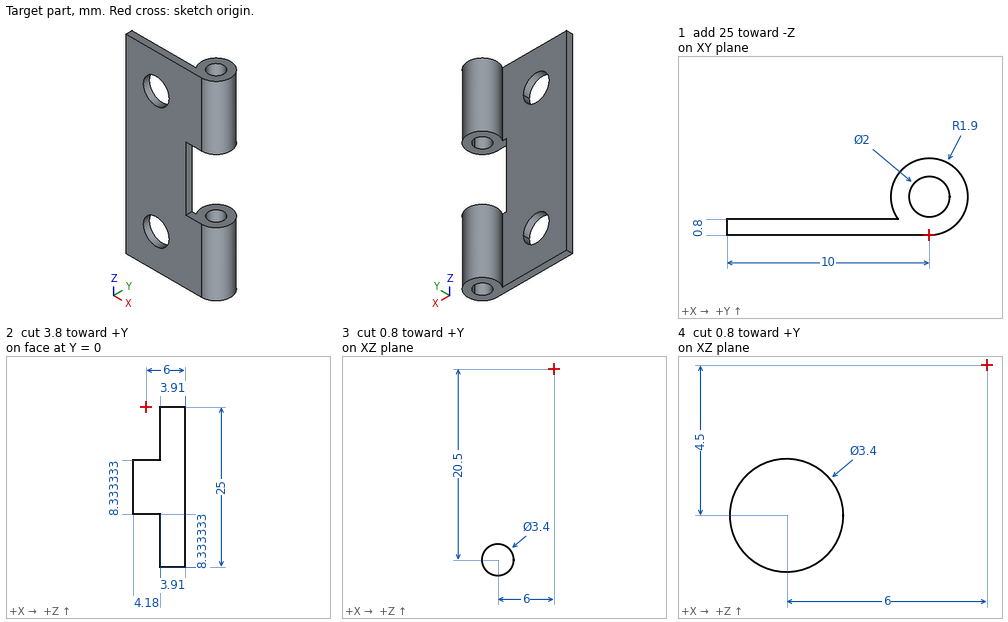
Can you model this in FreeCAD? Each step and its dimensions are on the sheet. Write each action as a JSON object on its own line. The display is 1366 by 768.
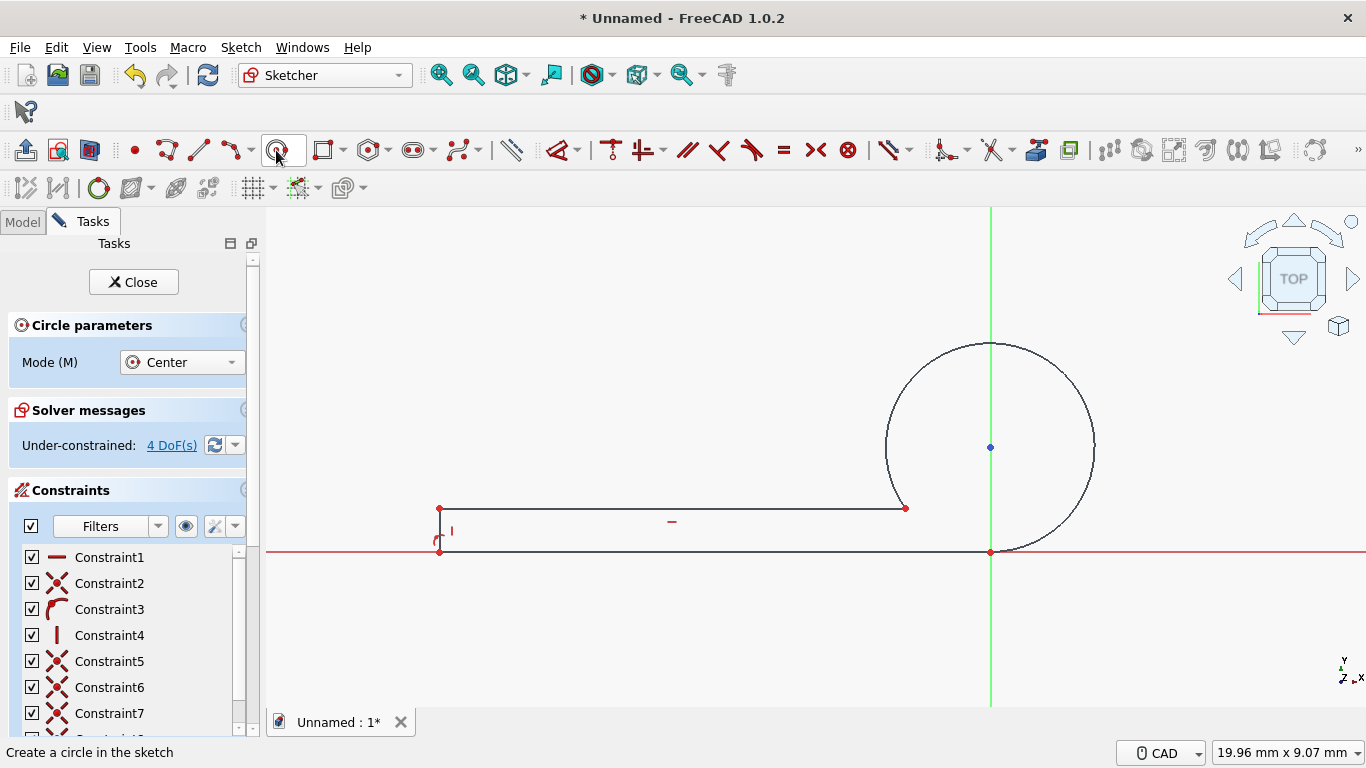
{"action": "left_click", "coordinate": [991, 447]}
{"action": "left_click", "coordinate": [1030, 408]}
{"action": "key", "text": "Escape"}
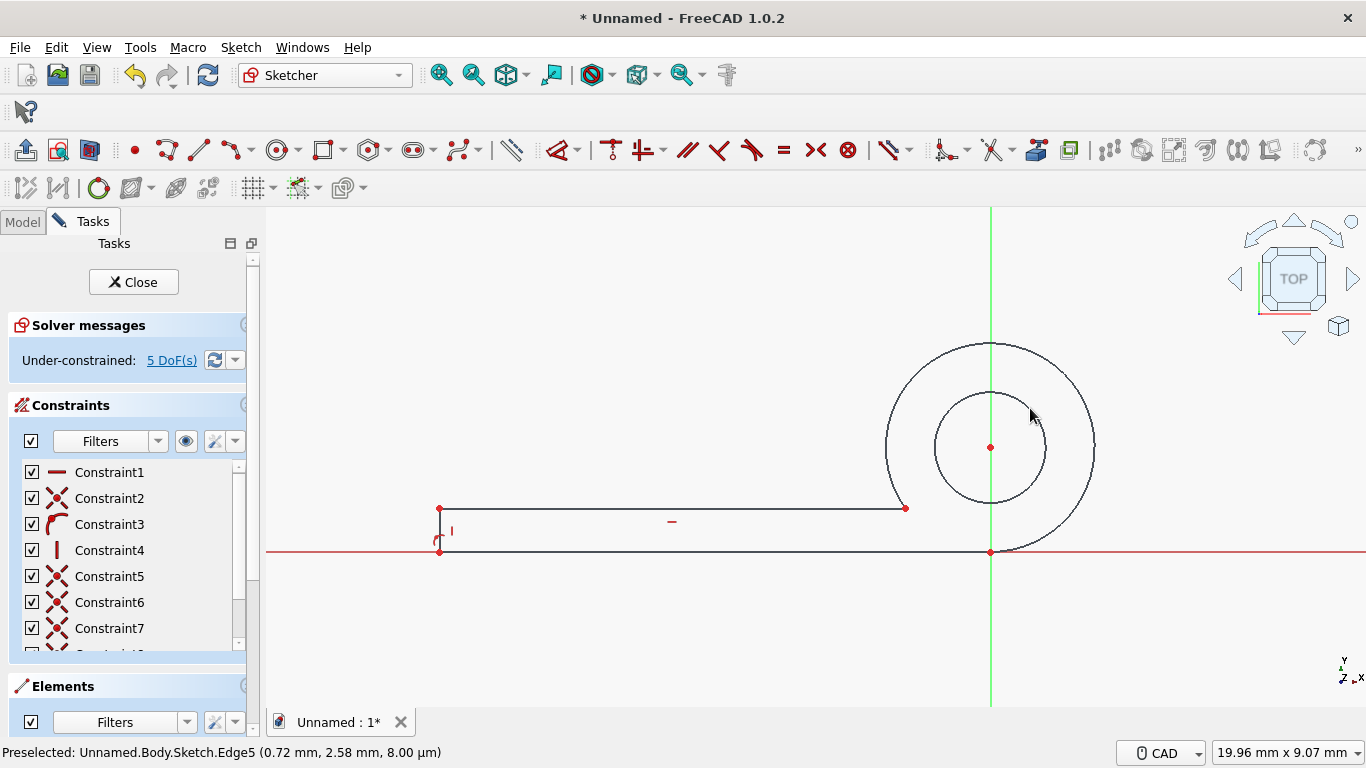
{"action": "left_click", "coordinate": [605, 552]}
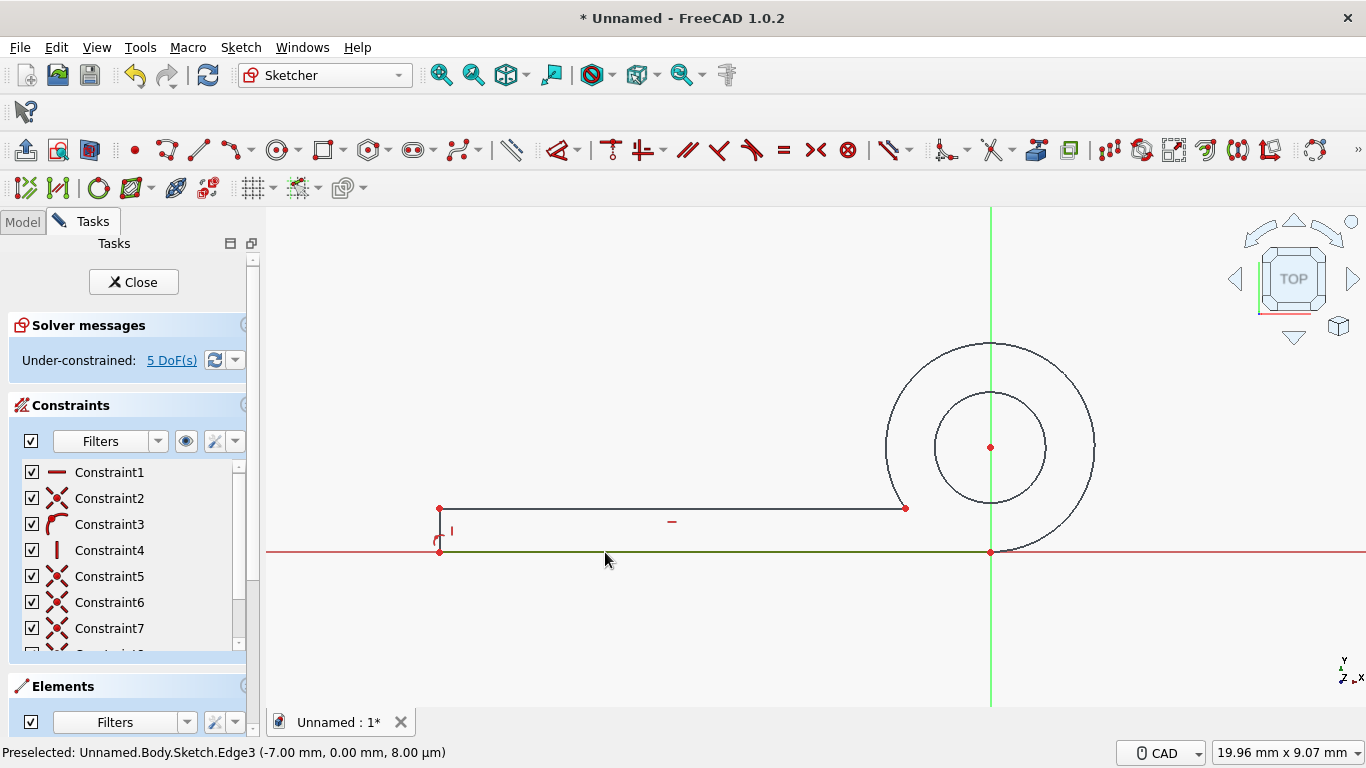
{"action": "left_click", "coordinate": [1095, 444]}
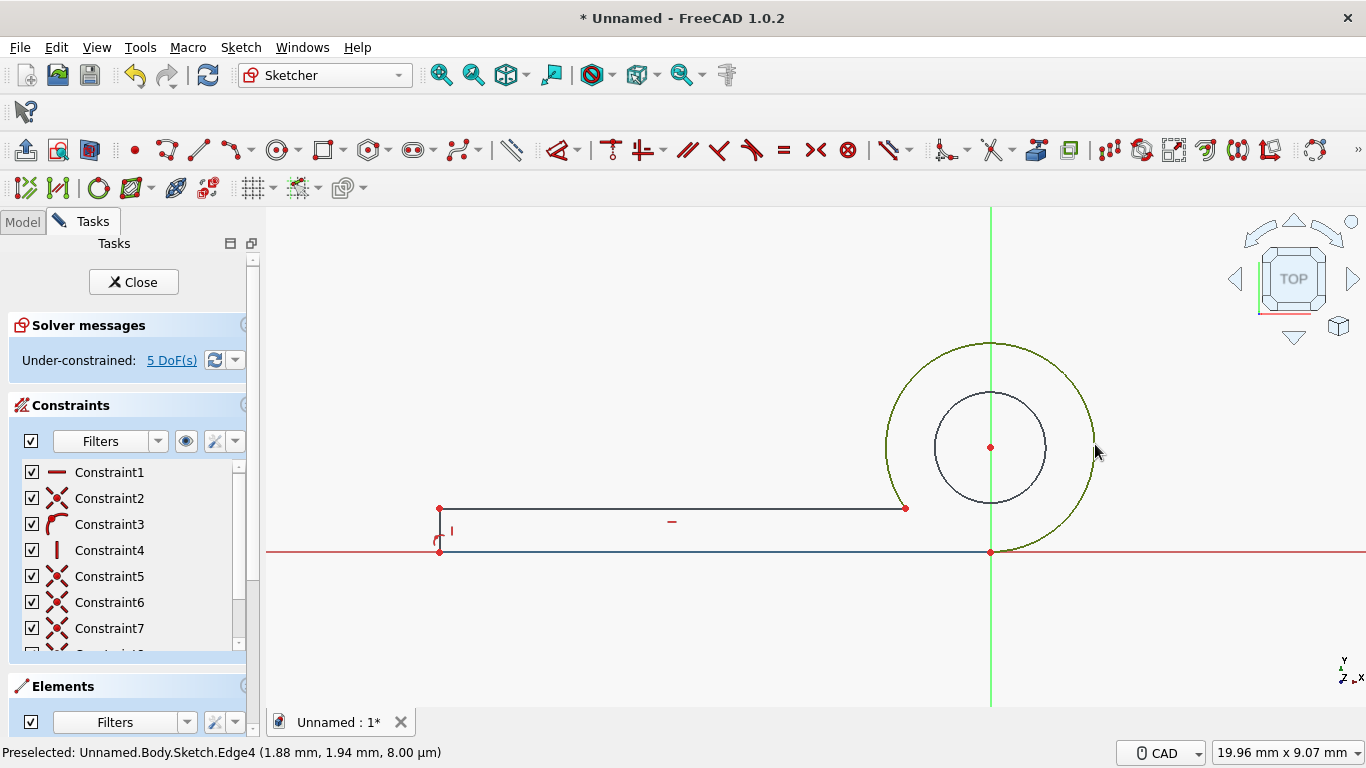
{"action": "left_click", "coordinate": [752, 150]}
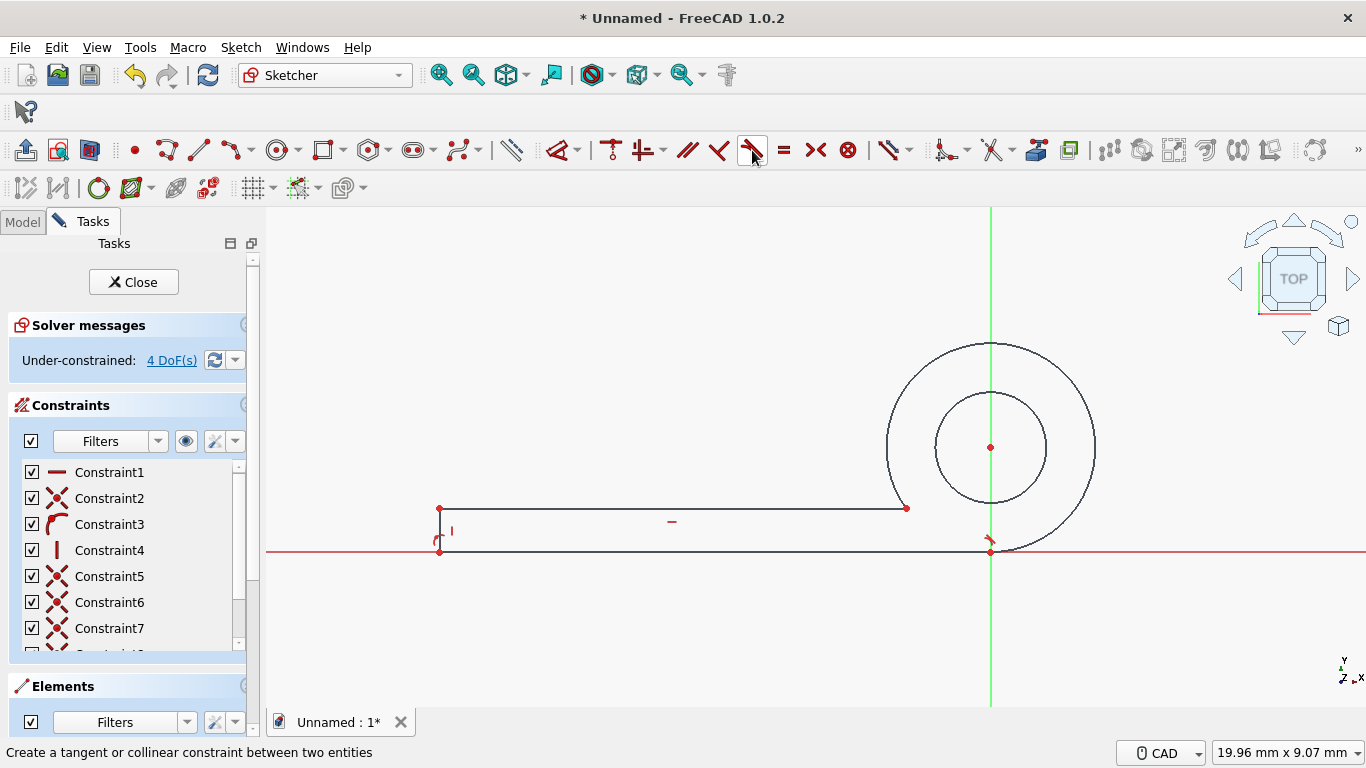
{"action": "left_click", "coordinate": [558, 150]}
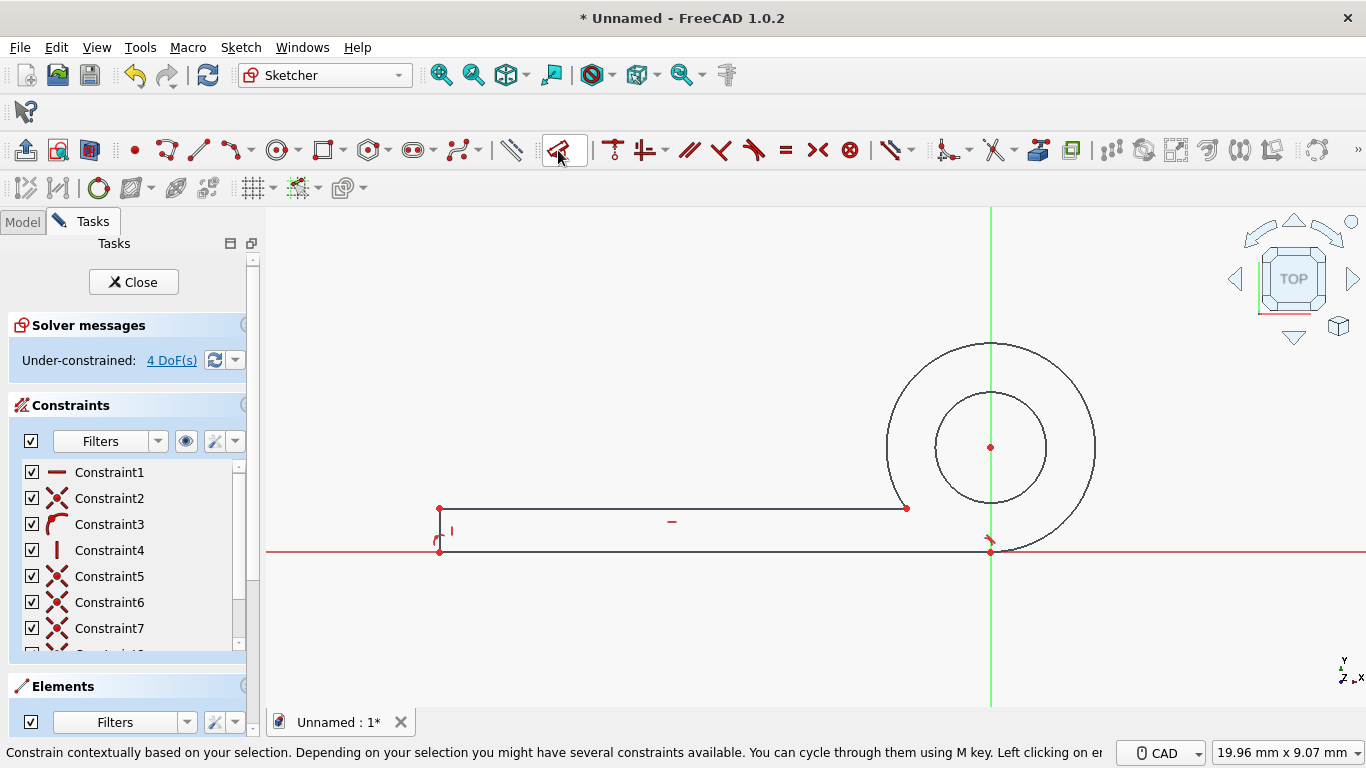
{"action": "left_click", "coordinate": [1095, 444]}
{"action": "left_click", "coordinate": [1127, 443]}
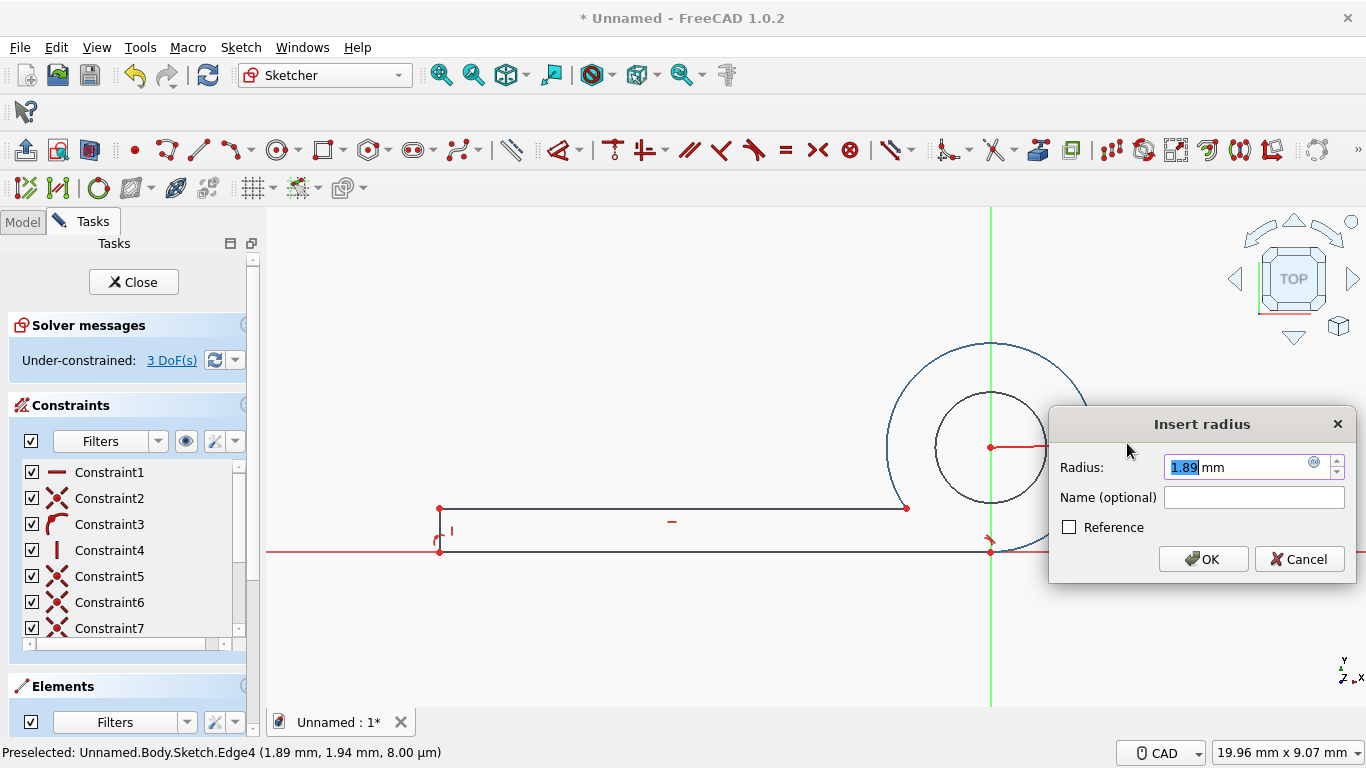
{"action": "type", "text": "1.9"}
{"action": "key", "text": "Return"}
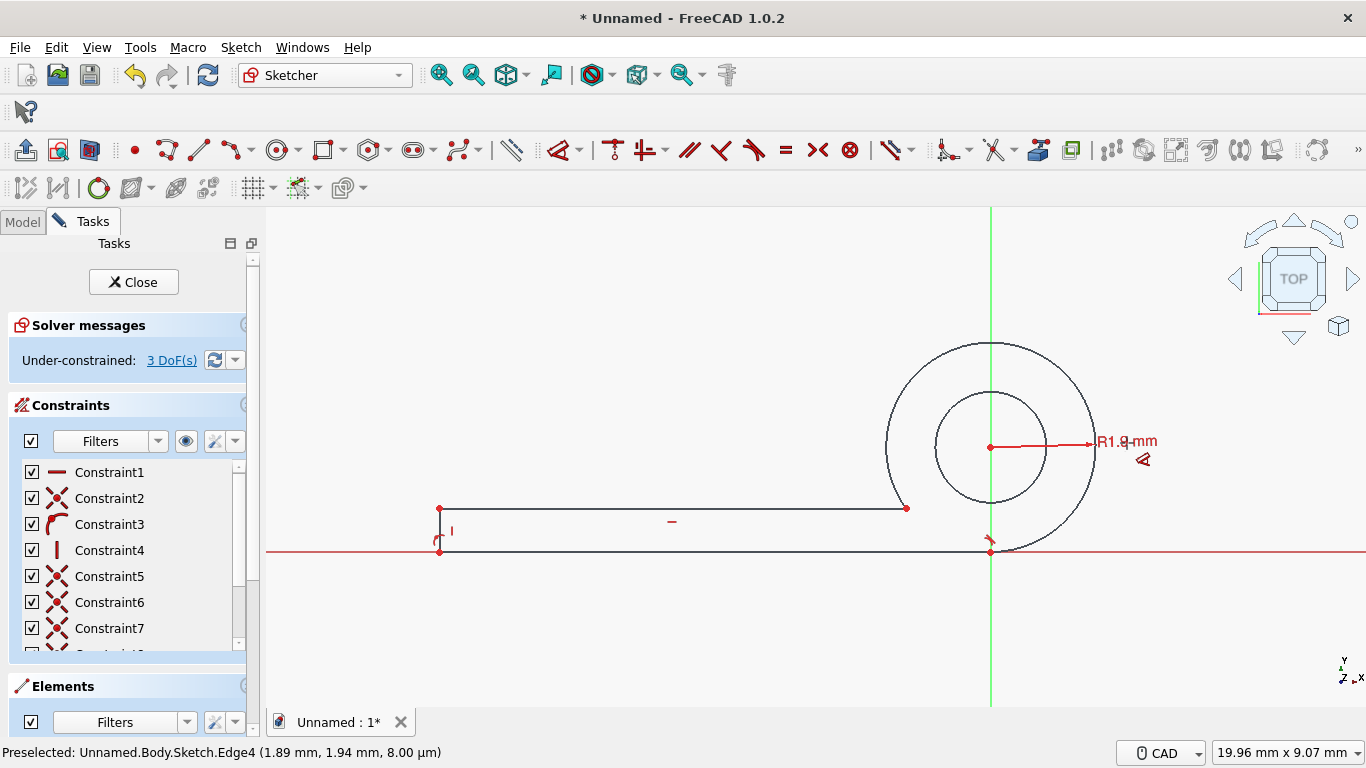
{"action": "left_click", "coordinate": [1030, 408]}
{"action": "left_click", "coordinate": [1053, 385]}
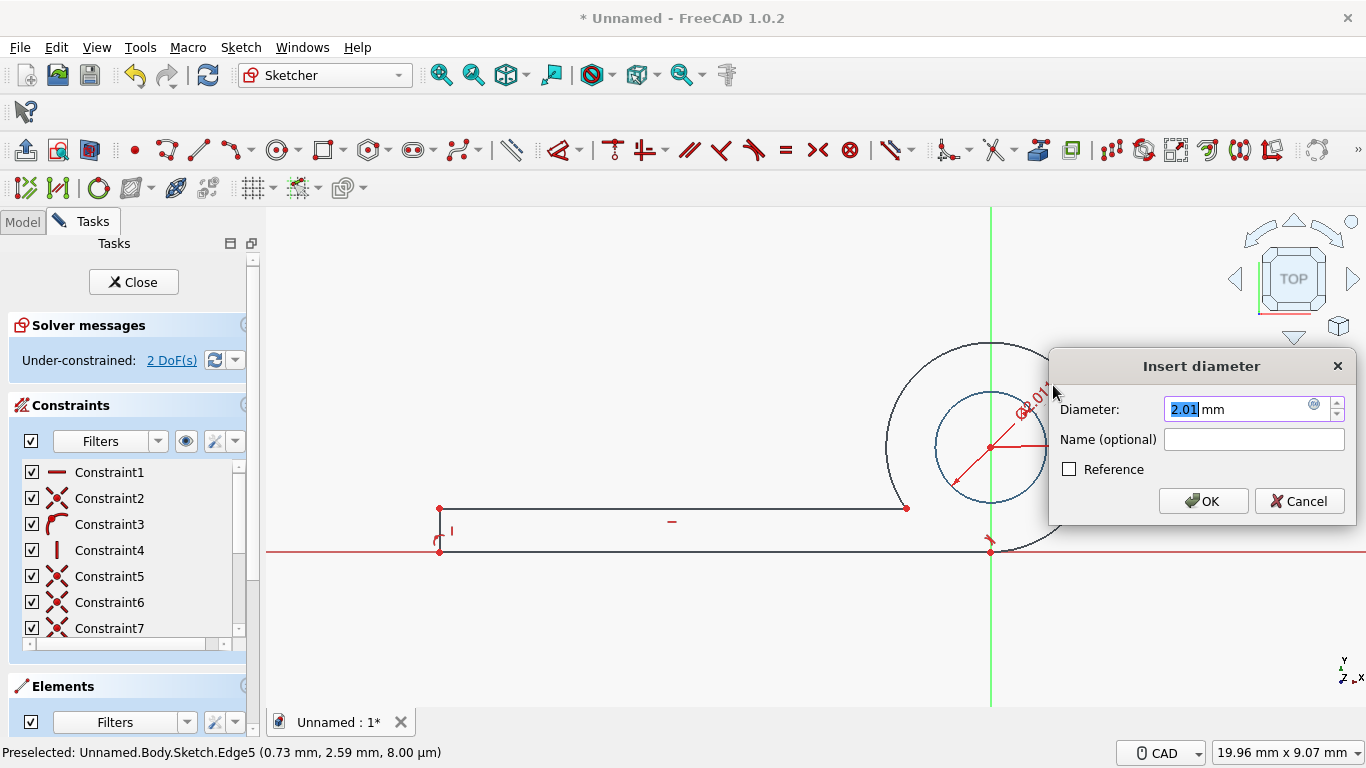
{"action": "type", "text": "2"}
{"action": "key", "text": "Return"}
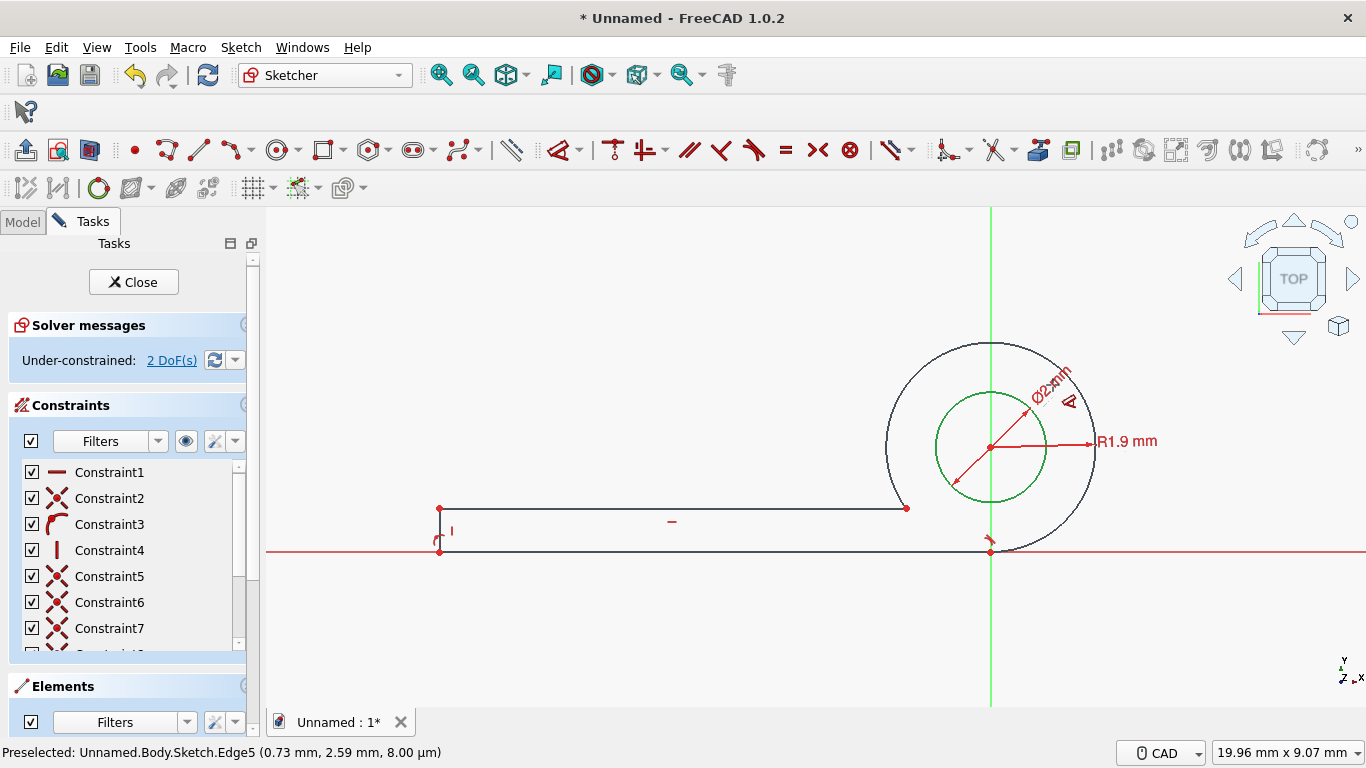
{"action": "left_click", "coordinate": [605, 552]}
{"action": "left_click", "coordinate": [715, 586]}